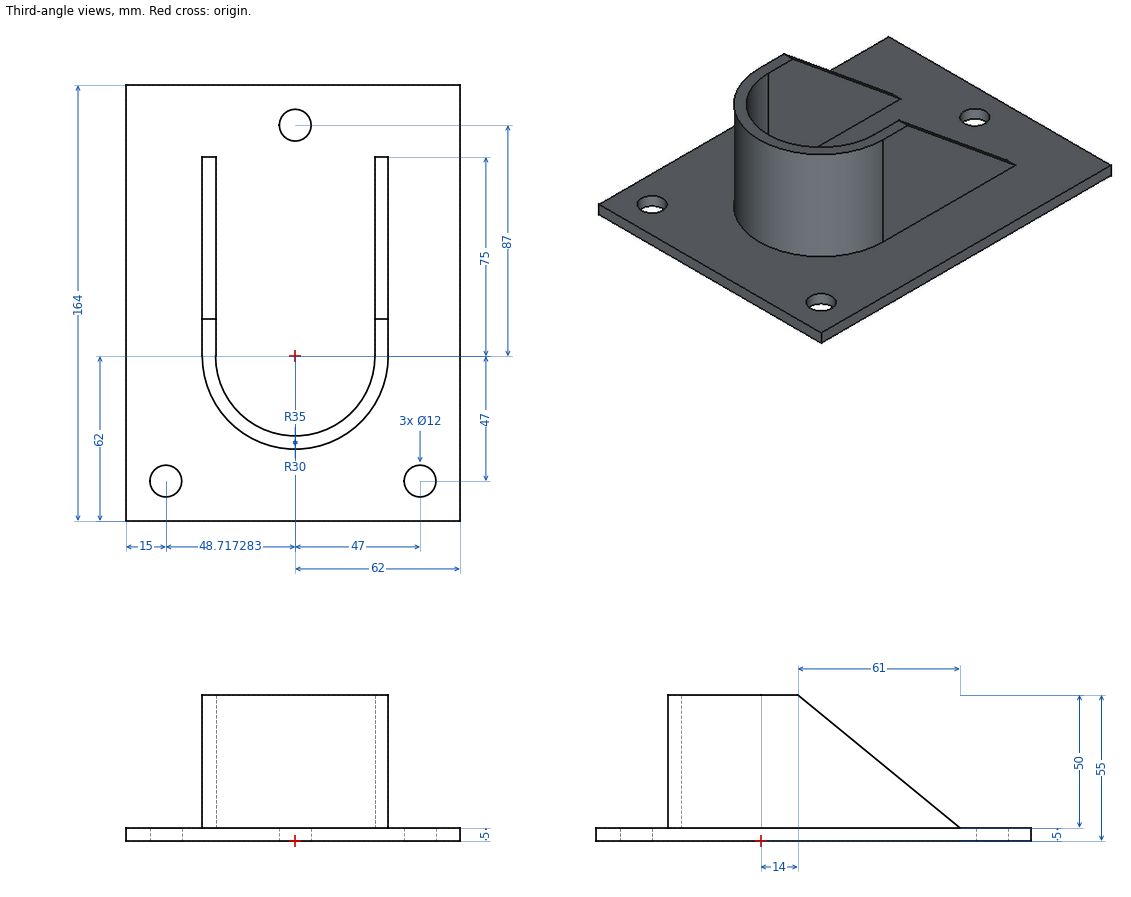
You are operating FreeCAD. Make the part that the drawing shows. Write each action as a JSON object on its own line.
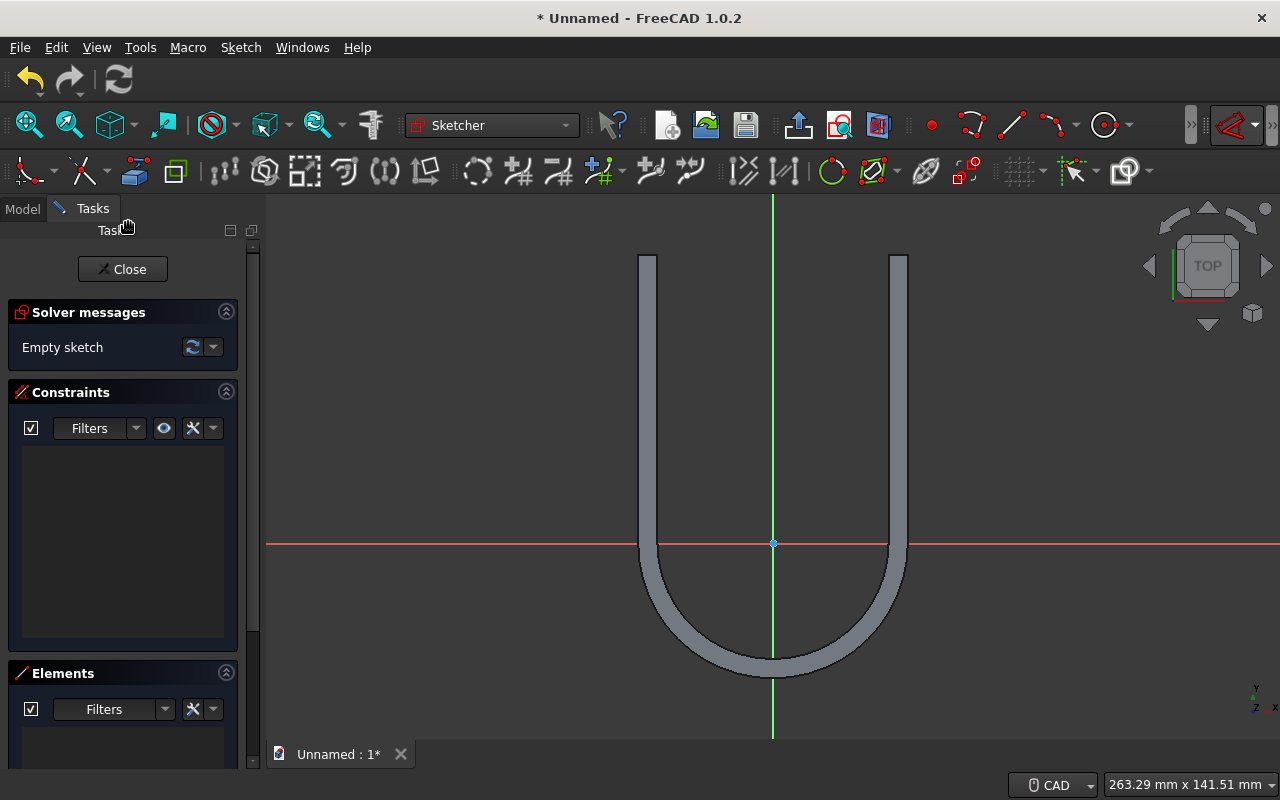
{"action": "left_click", "coordinate": [880, 126]}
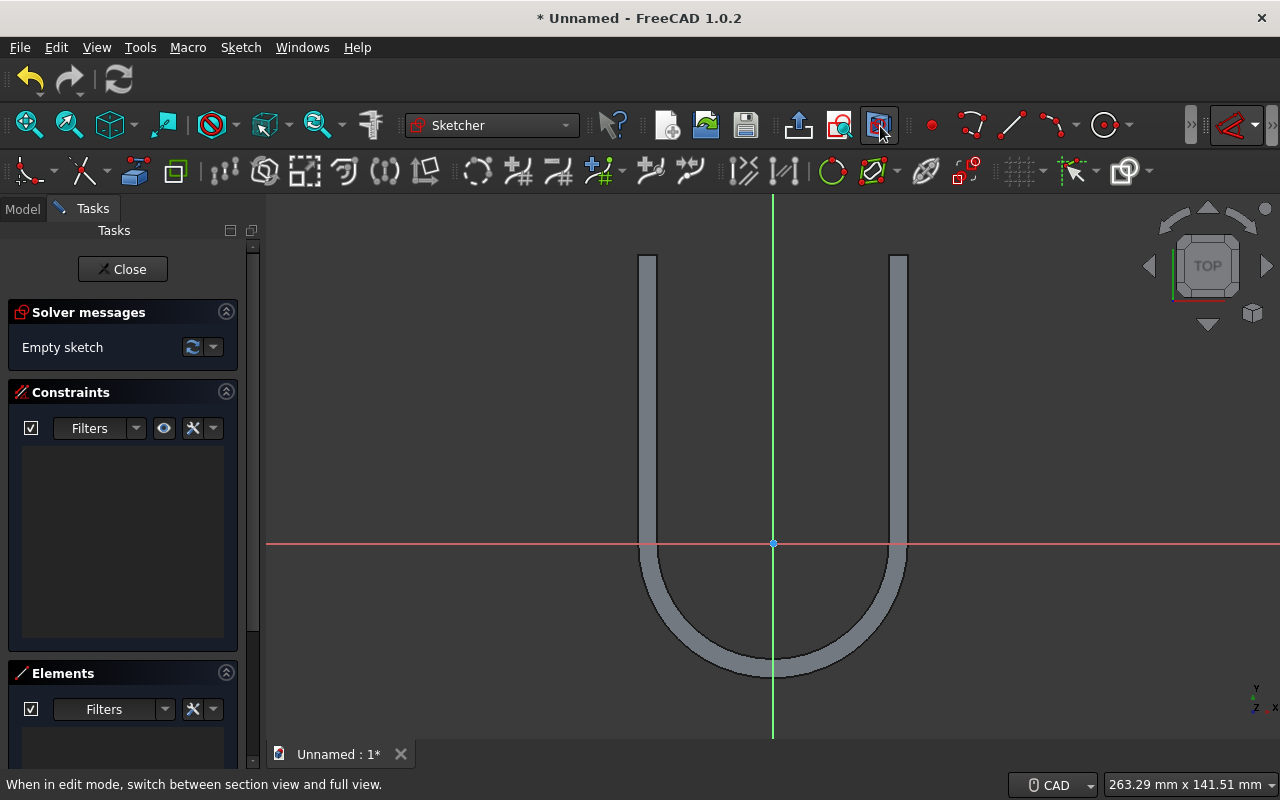
{"action": "scroll", "coordinate": [625, 466], "scroll_direction": "down", "scroll_amount": 3}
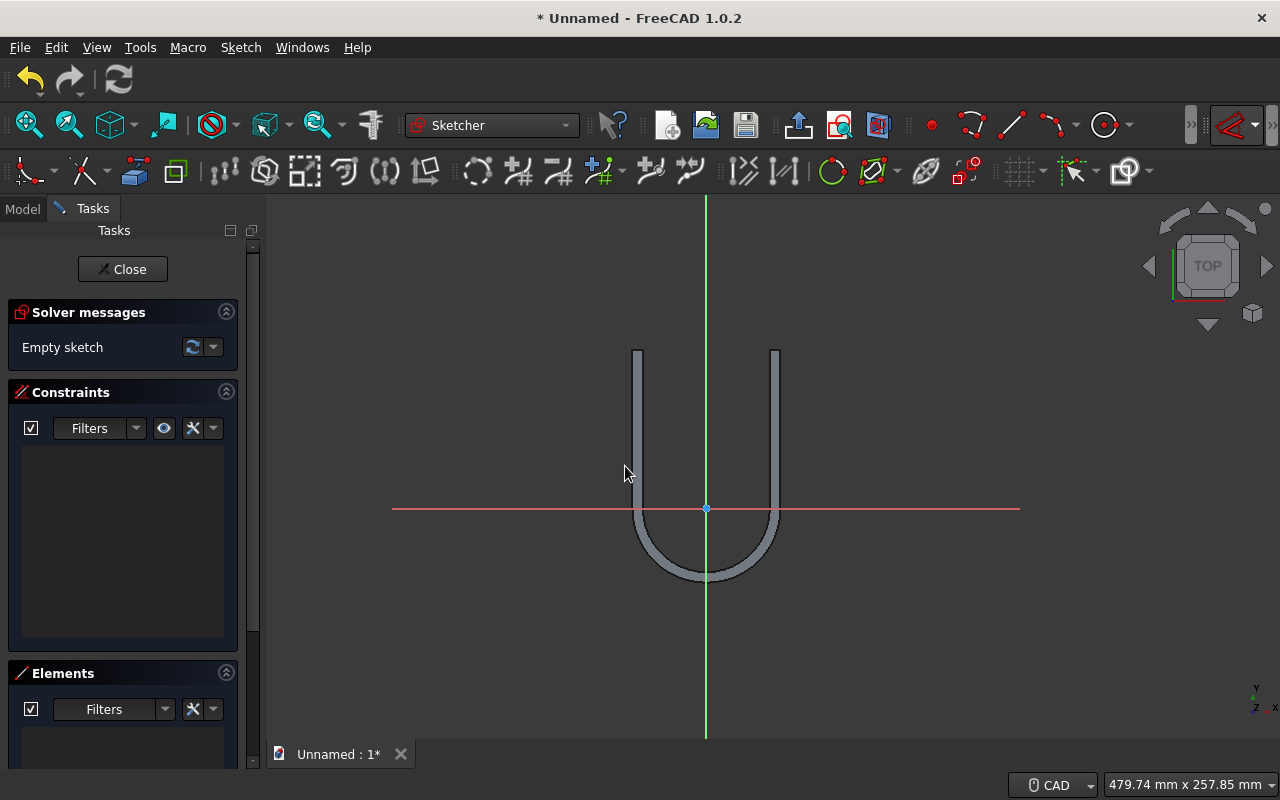
{"action": "key", "text": "g r"}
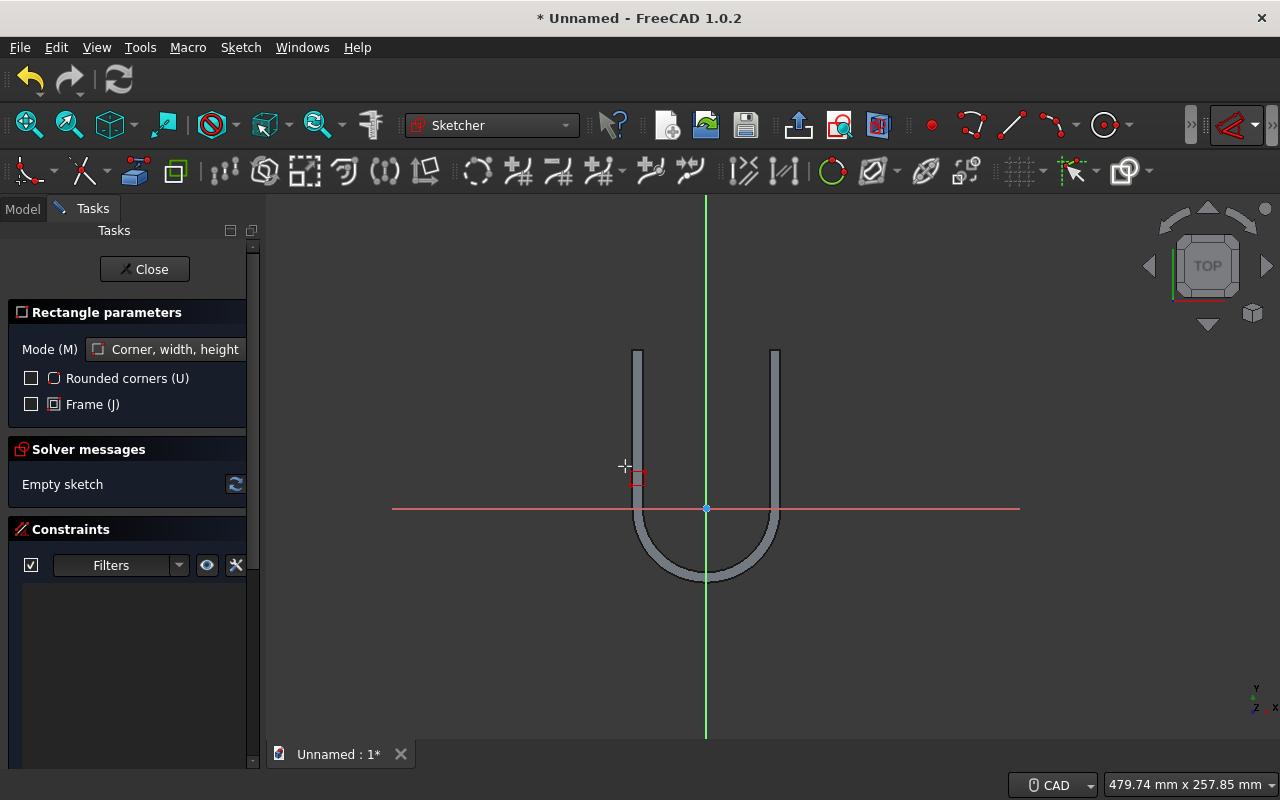
{"action": "left_click", "coordinate": [572, 293]}
{"action": "left_click", "coordinate": [837, 640]}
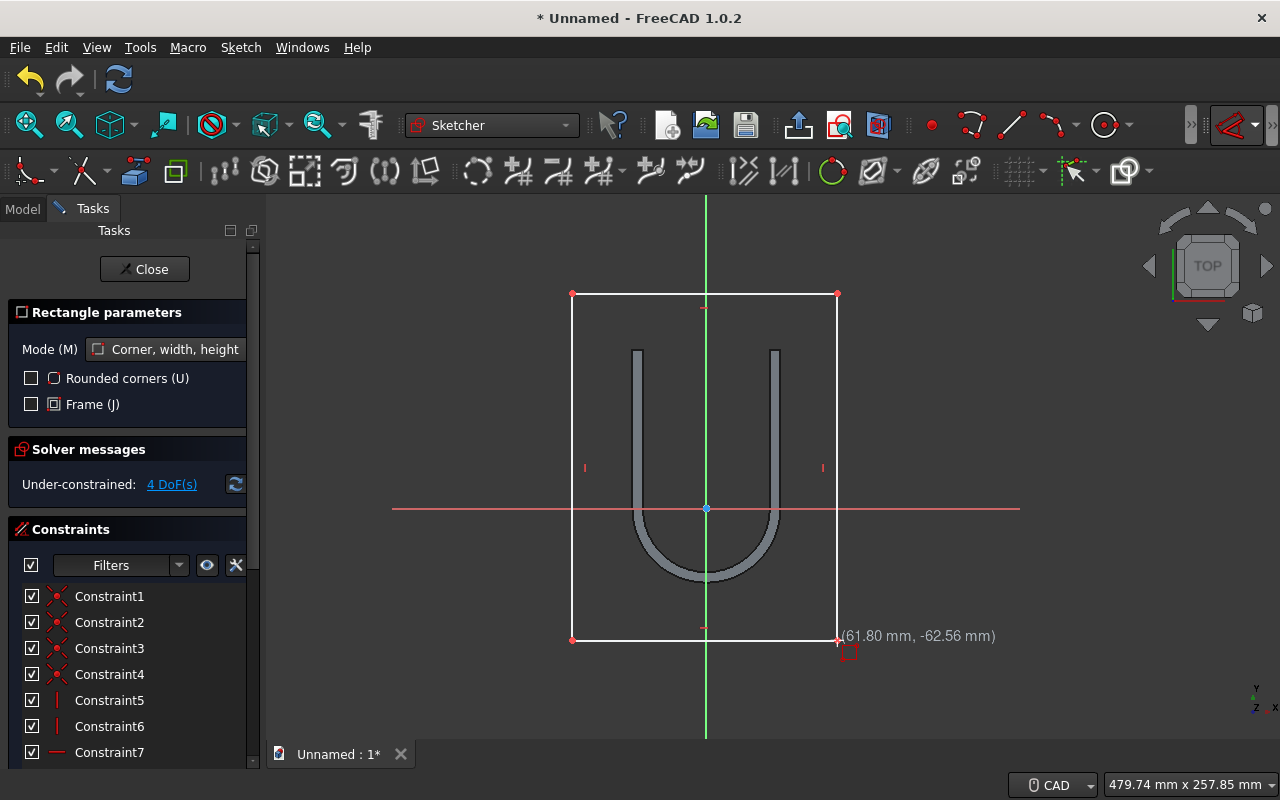
{"action": "left_click", "coordinate": [1106, 126]}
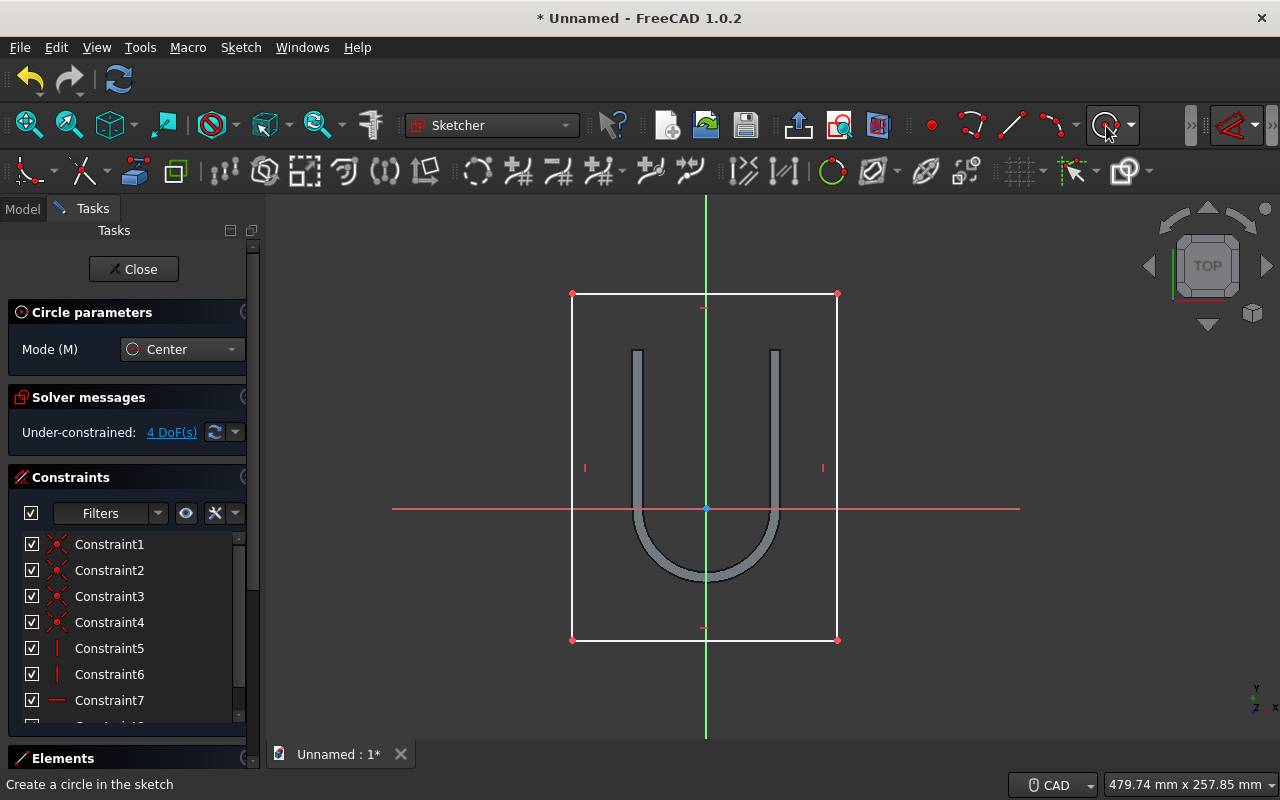
{"action": "scroll", "coordinate": [806, 608], "scroll_direction": "up", "scroll_amount": 3}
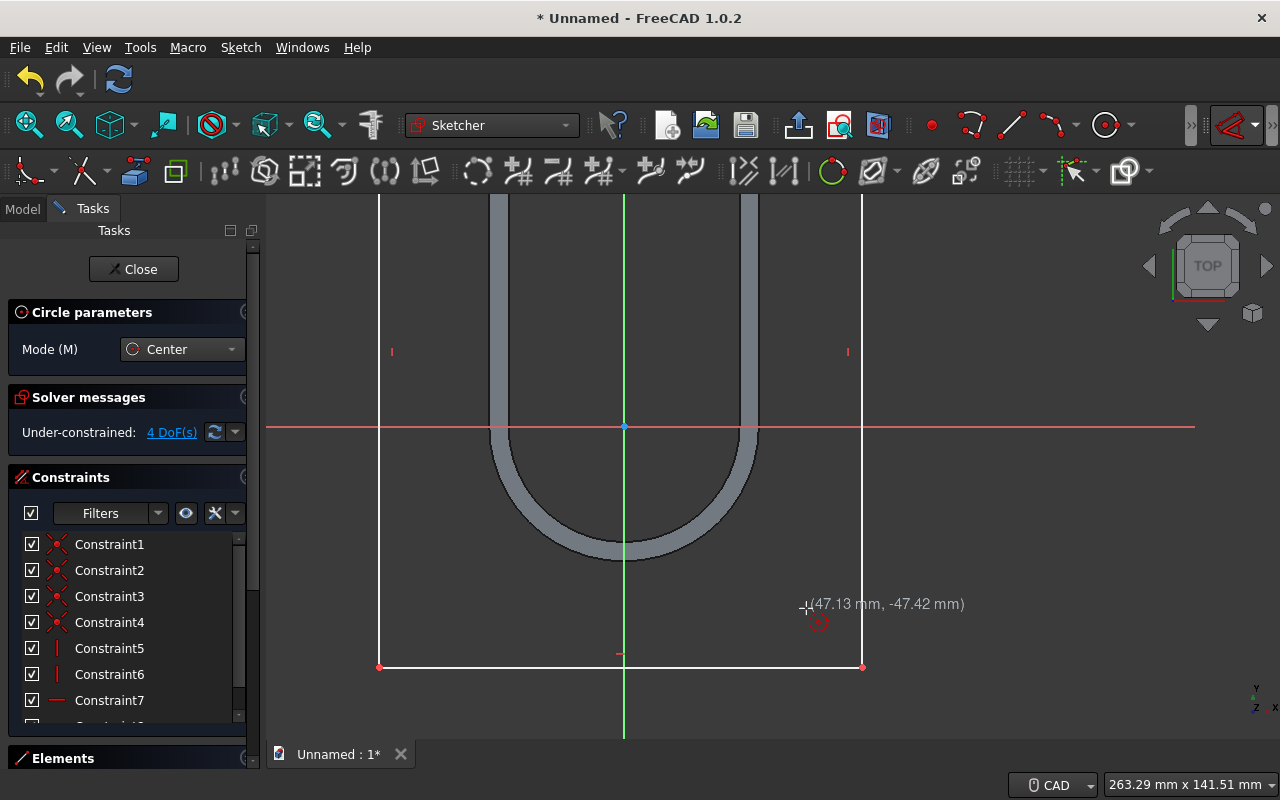
{"action": "left_click", "coordinate": [805, 608]}
{"action": "left_click", "coordinate": [821, 591]}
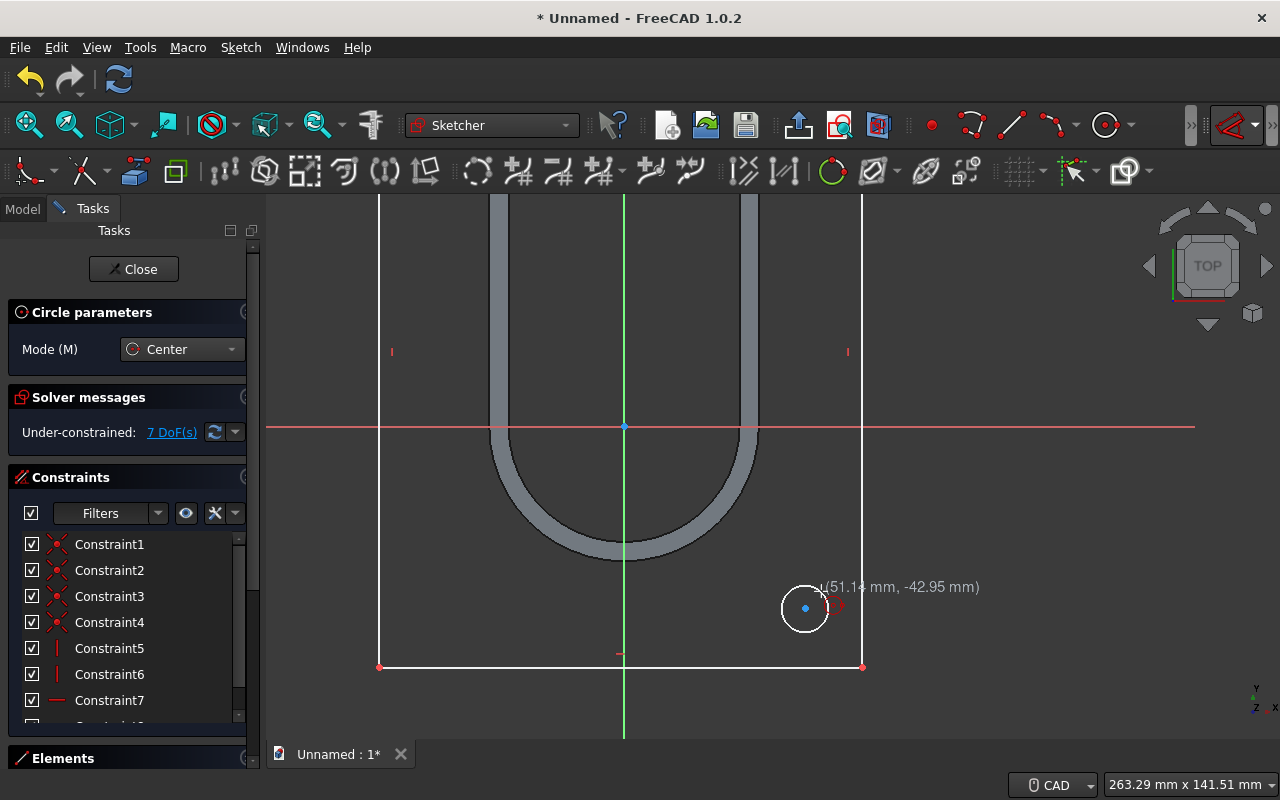
{"action": "left_click", "coordinate": [436, 608]}
{"action": "left_click", "coordinate": [453, 591]}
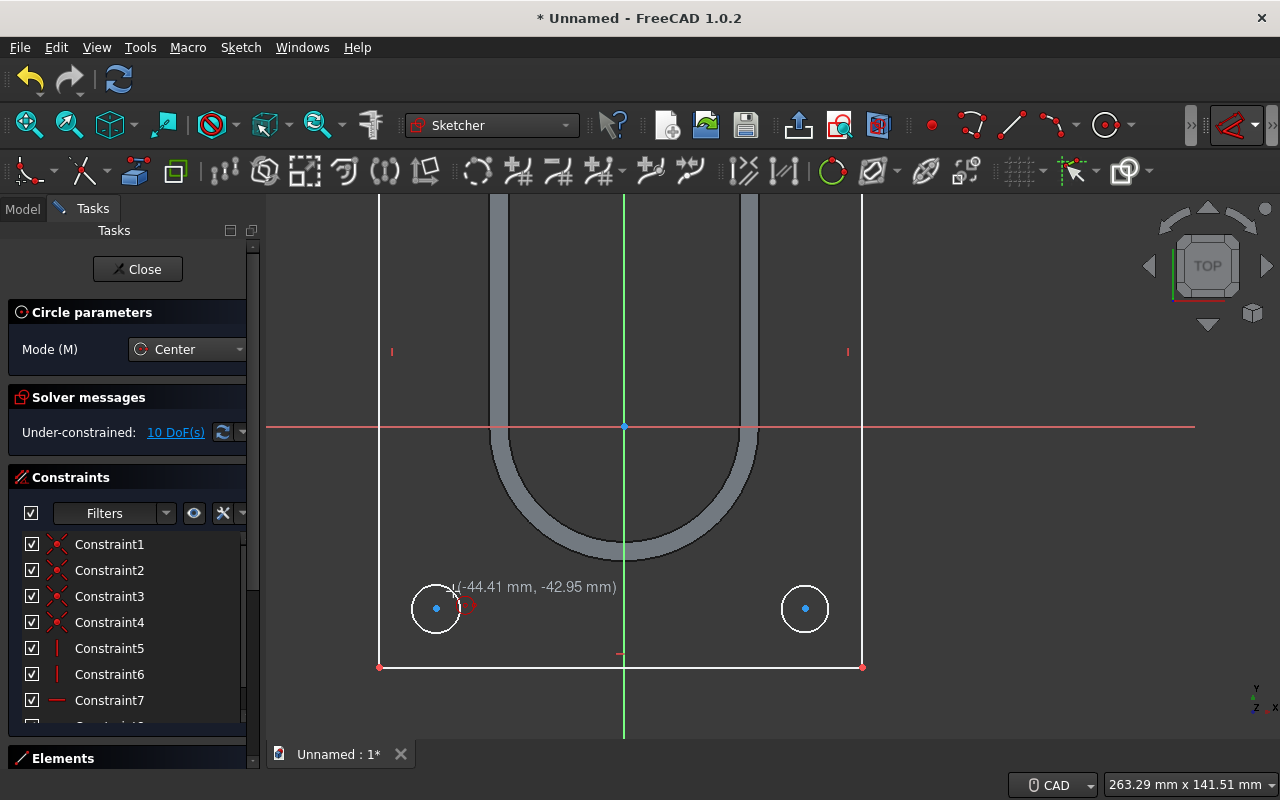
{"action": "scroll", "coordinate": [806, 609], "scroll_direction": "down", "scroll_amount": 3}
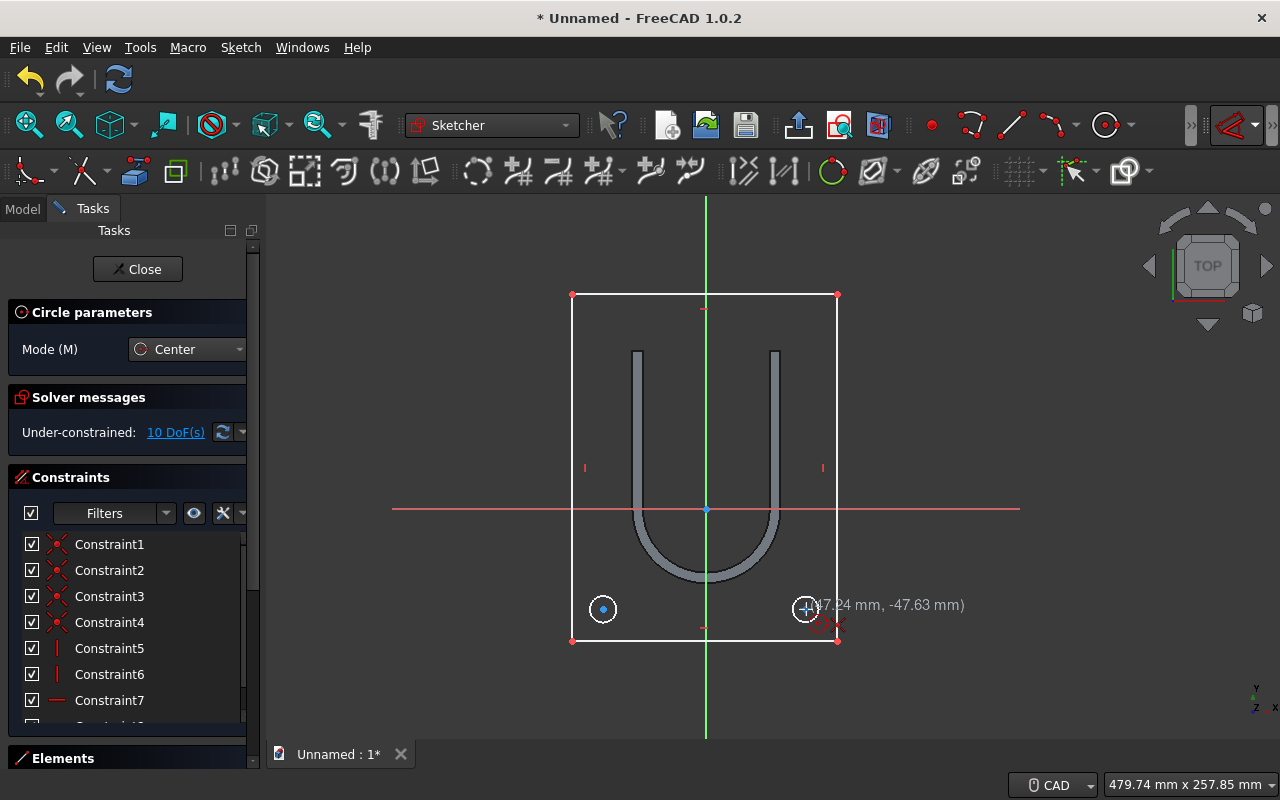
{"action": "scroll", "coordinate": [706, 325], "scroll_direction": "up", "scroll_amount": 3}